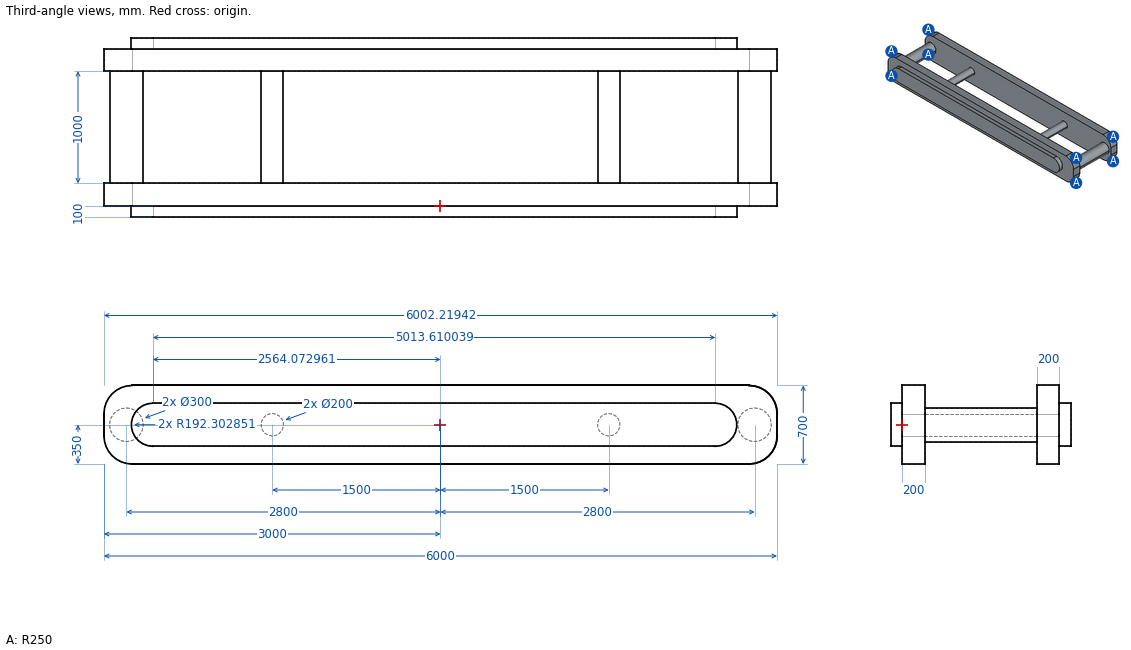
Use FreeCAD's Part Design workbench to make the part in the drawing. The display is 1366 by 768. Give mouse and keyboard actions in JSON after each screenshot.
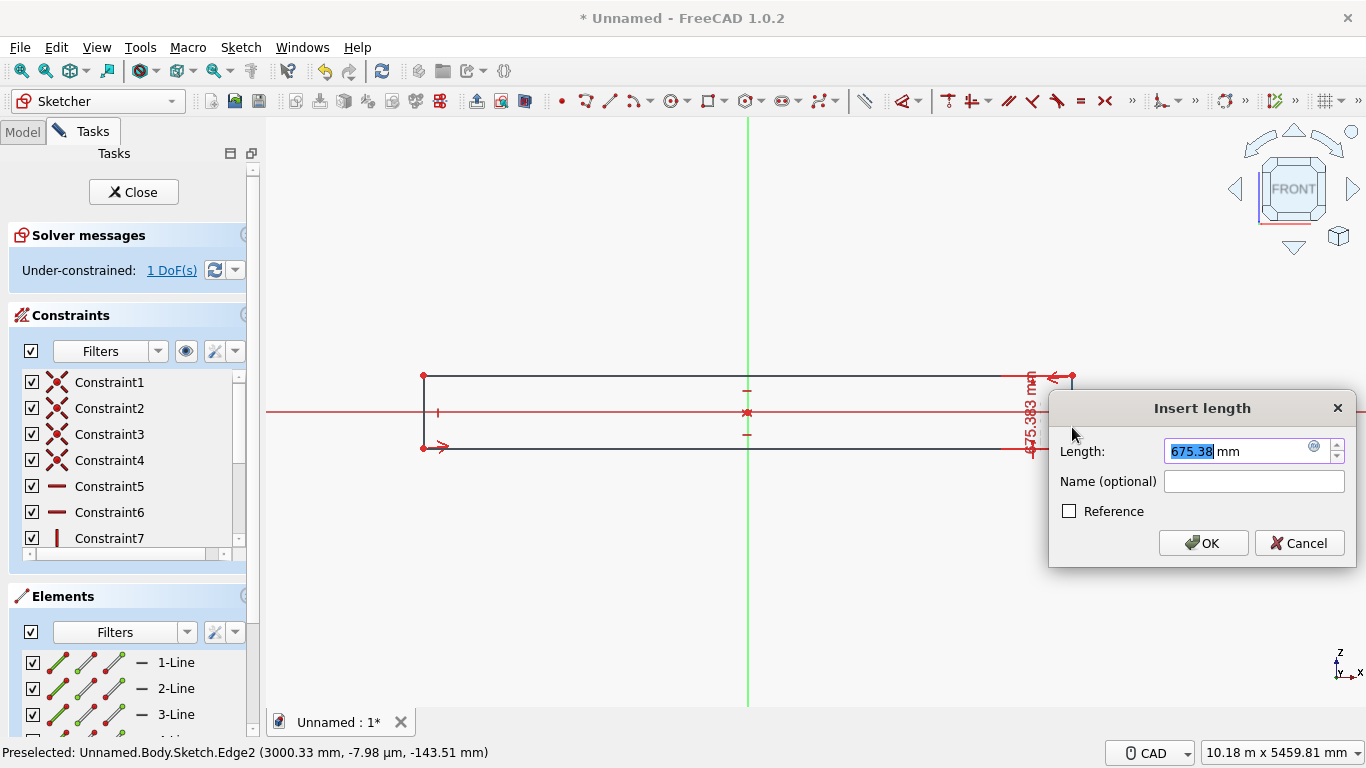
{"action": "type", "text": "700"}
{"action": "key", "text": "Return"}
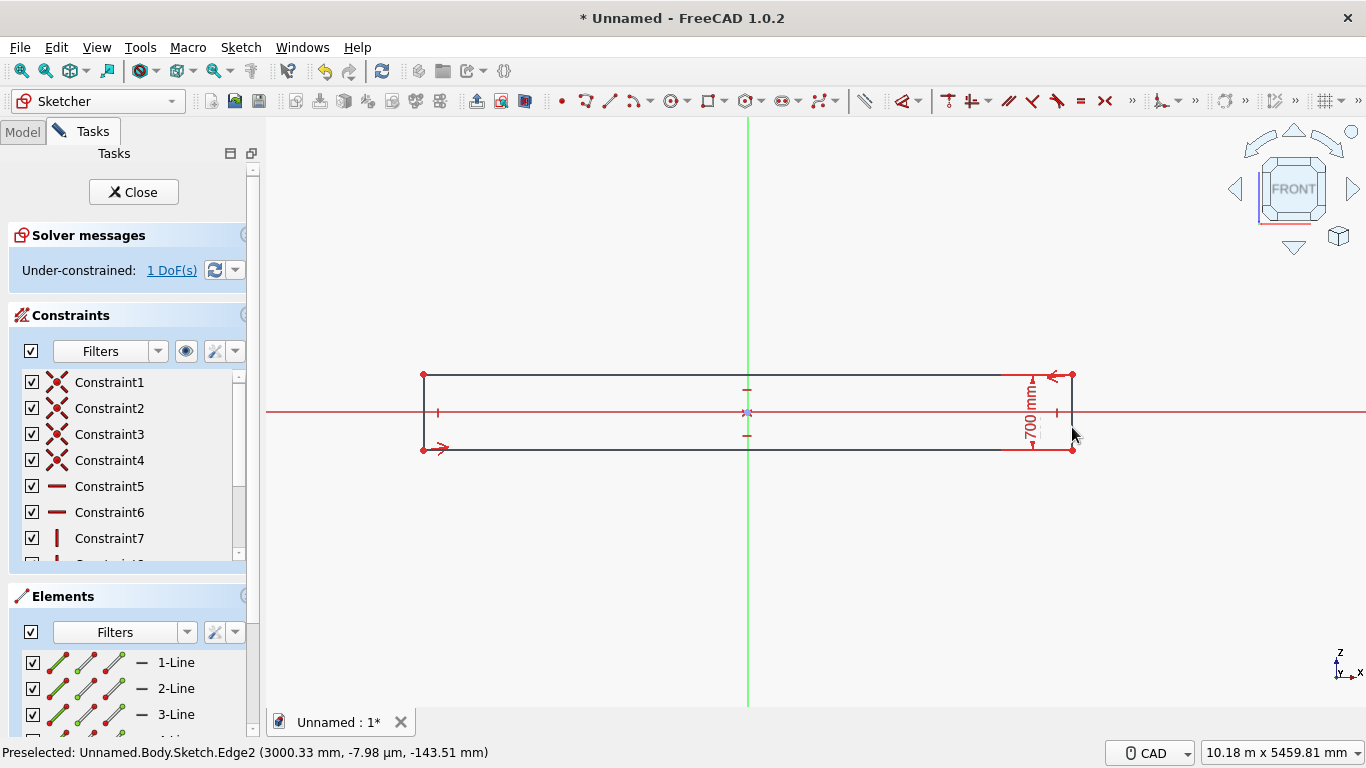
{"action": "left_click", "coordinate": [618, 450]}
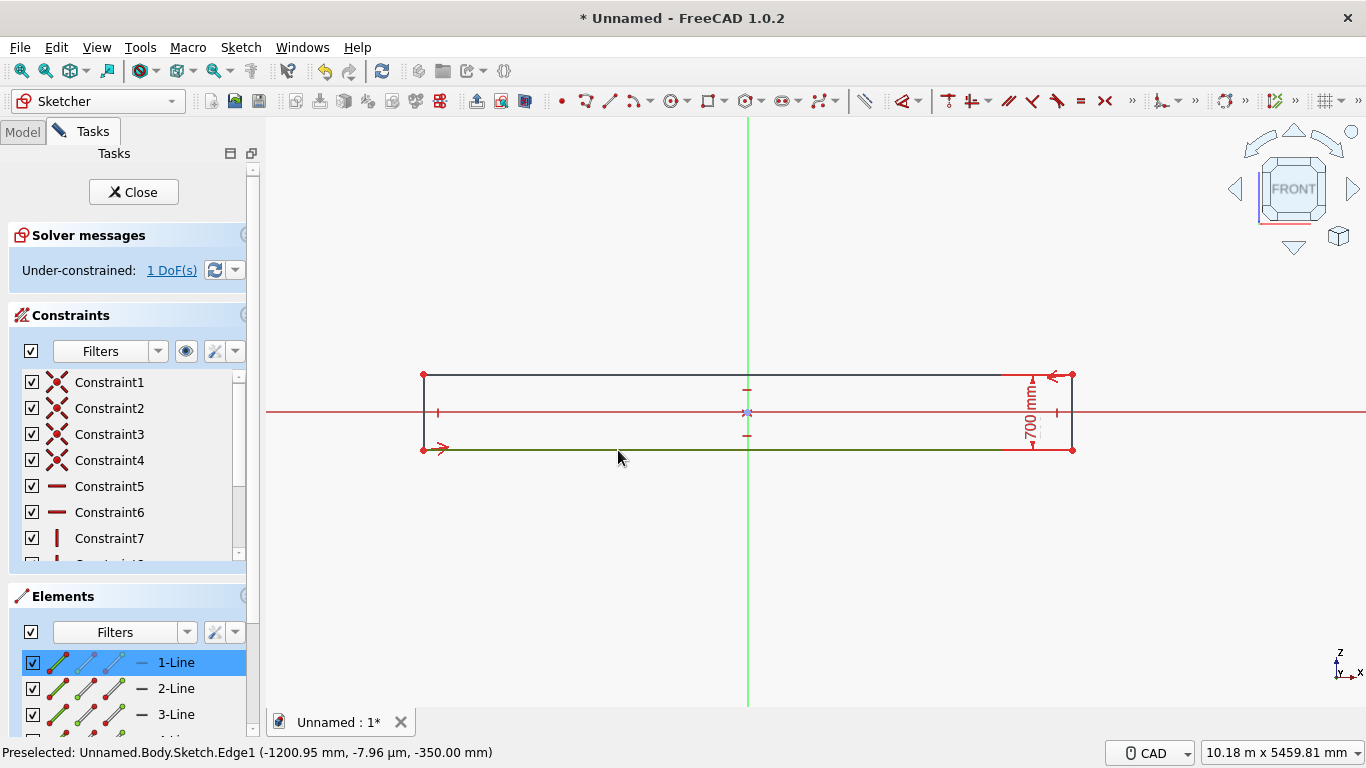
{"action": "key", "text": "l"}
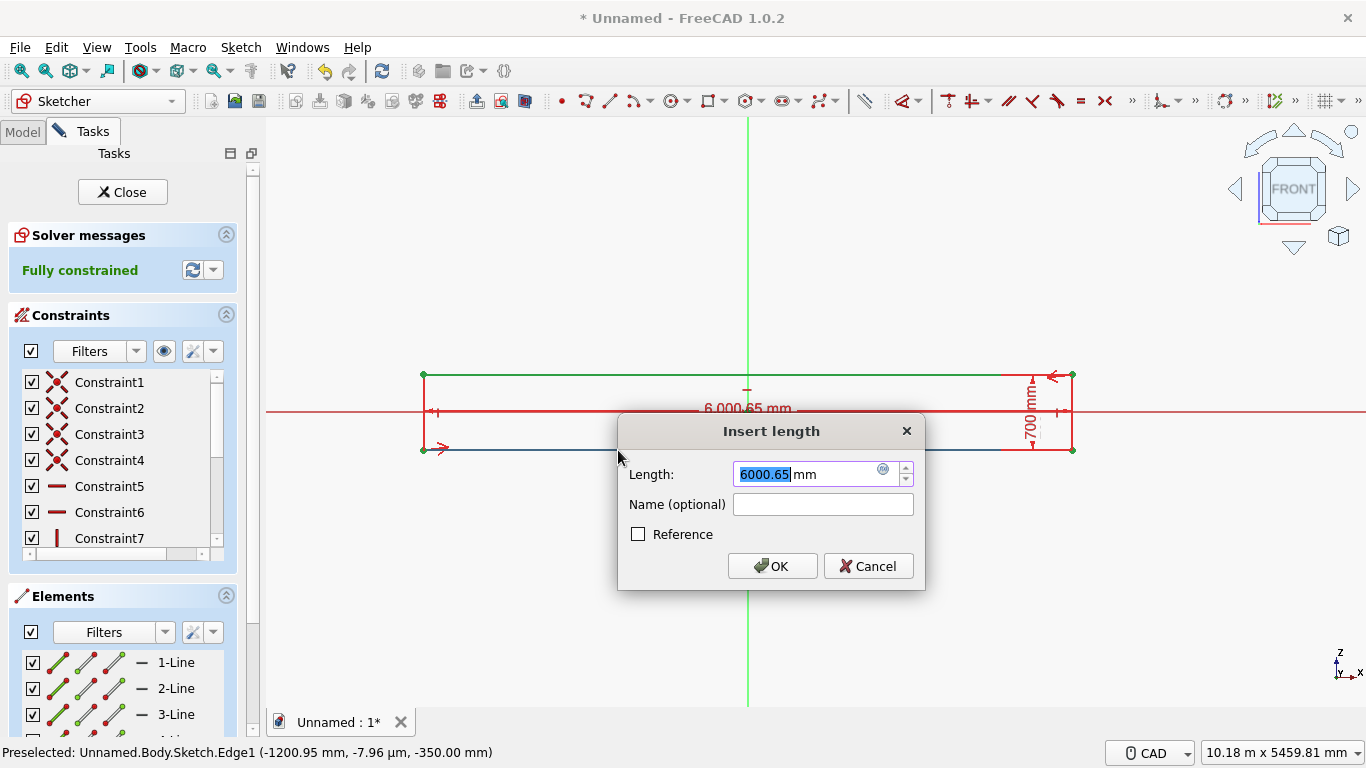
{"action": "type", "text": "6000"}
{"action": "key", "text": "Return"}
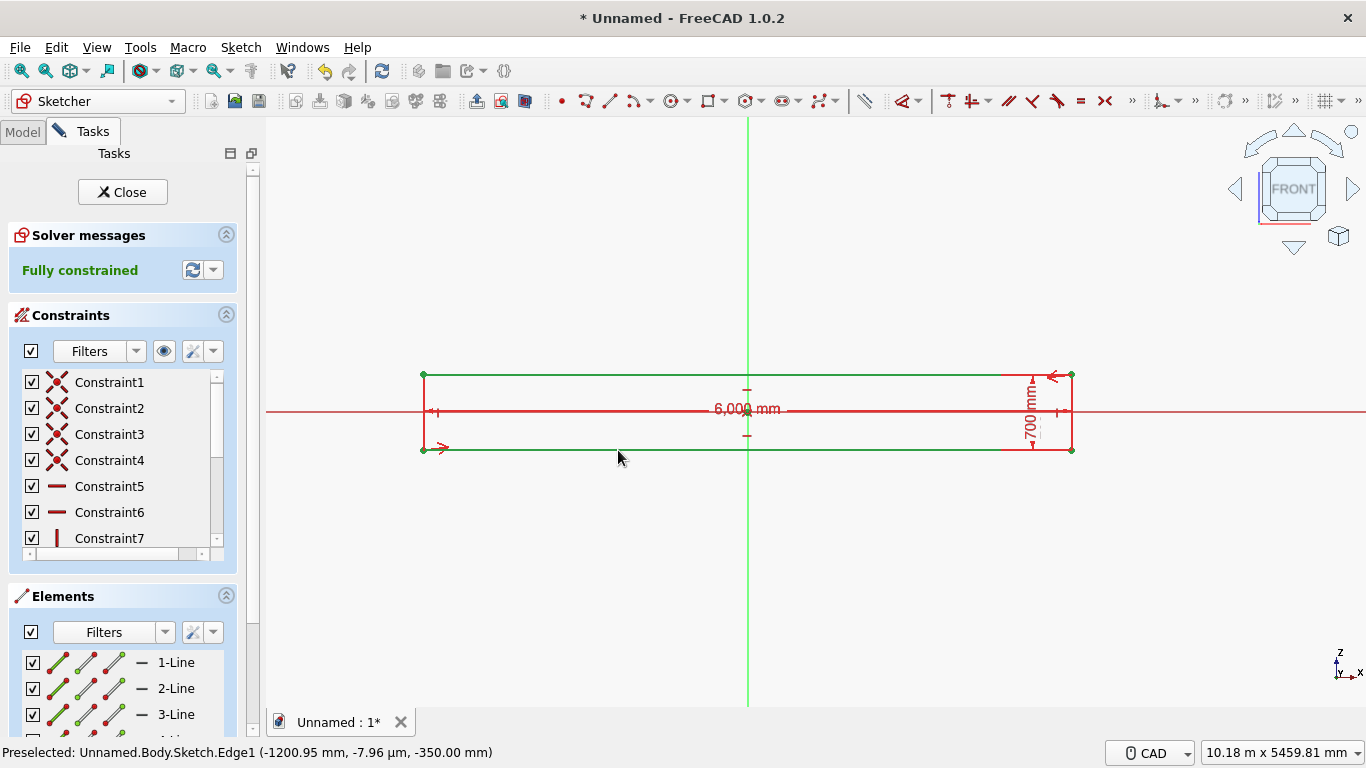
{"action": "left_click", "coordinate": [123, 192]}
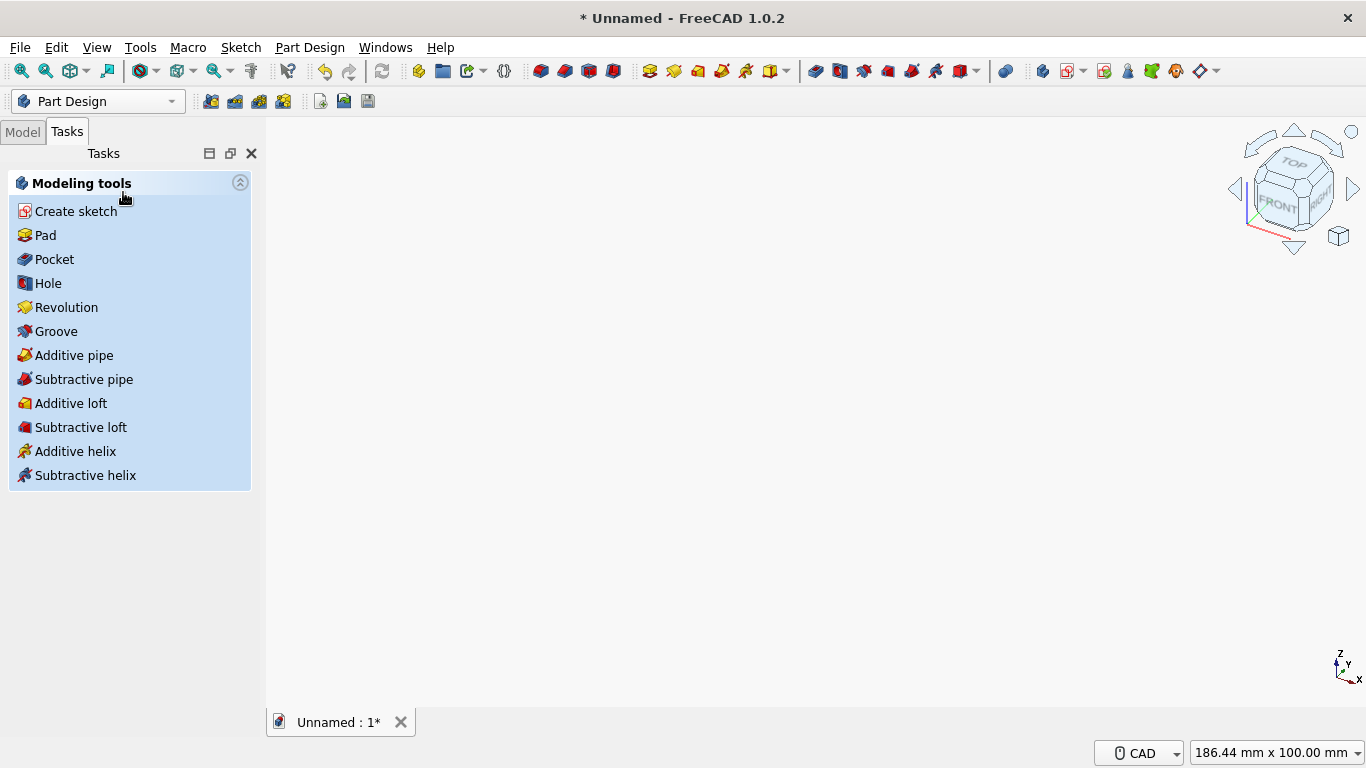
{"action": "left_click", "coordinate": [650, 72]}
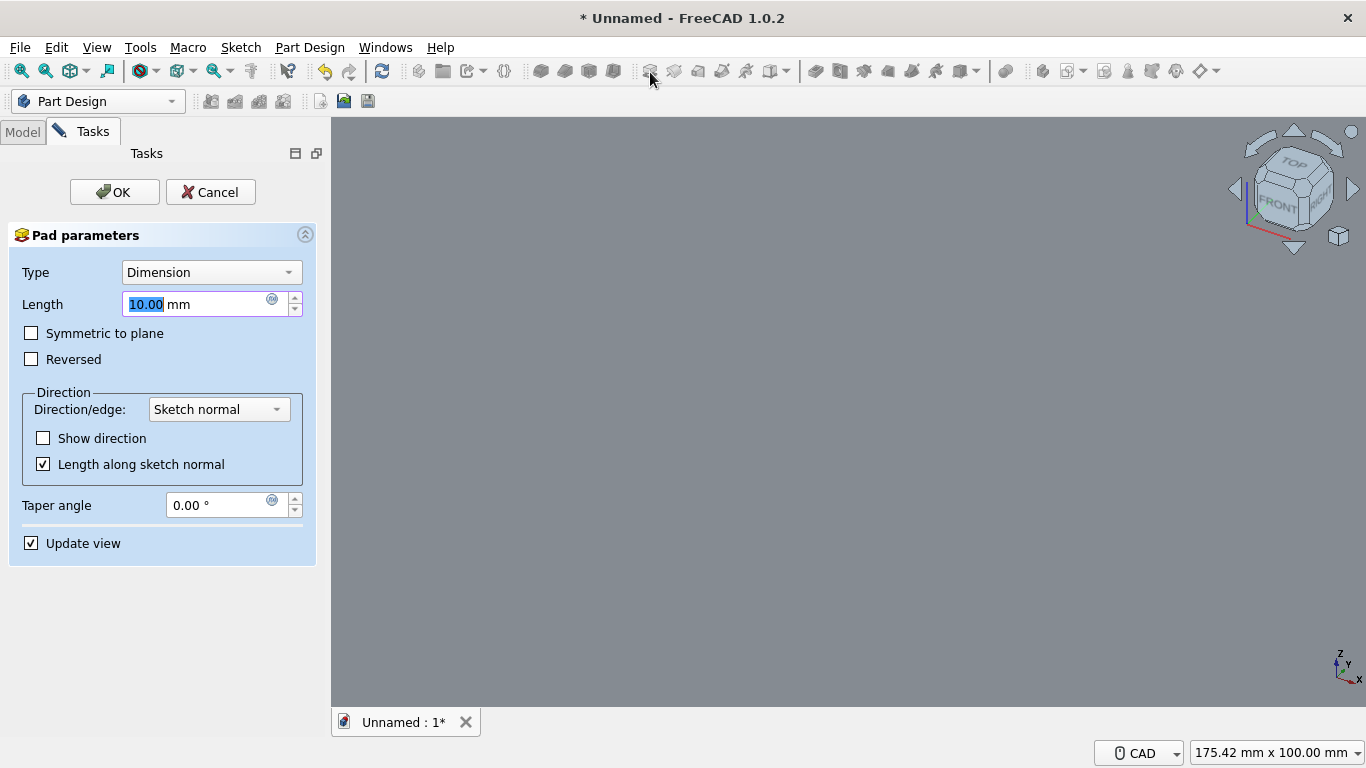
{"action": "type", "text": "200"}
{"action": "key", "text": "Tab"}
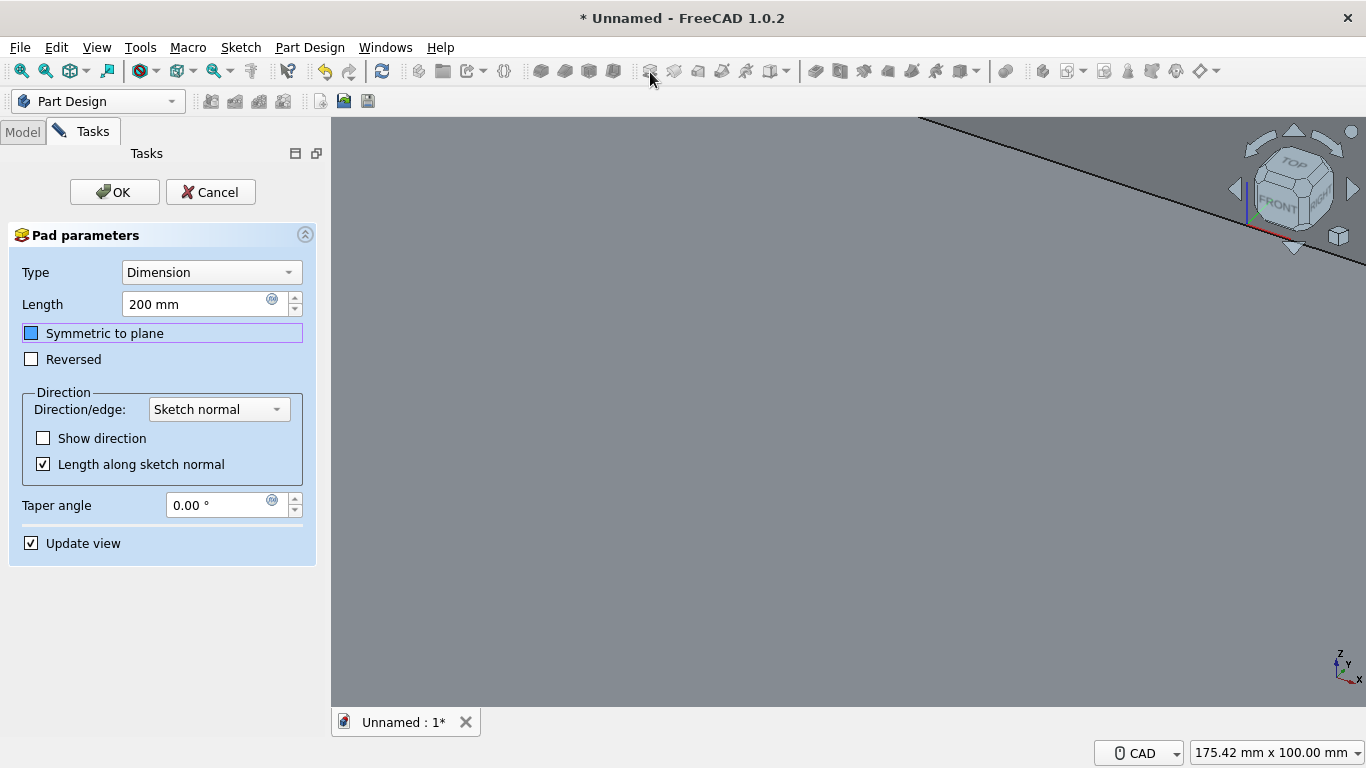
{"action": "left_click", "coordinate": [30, 359]}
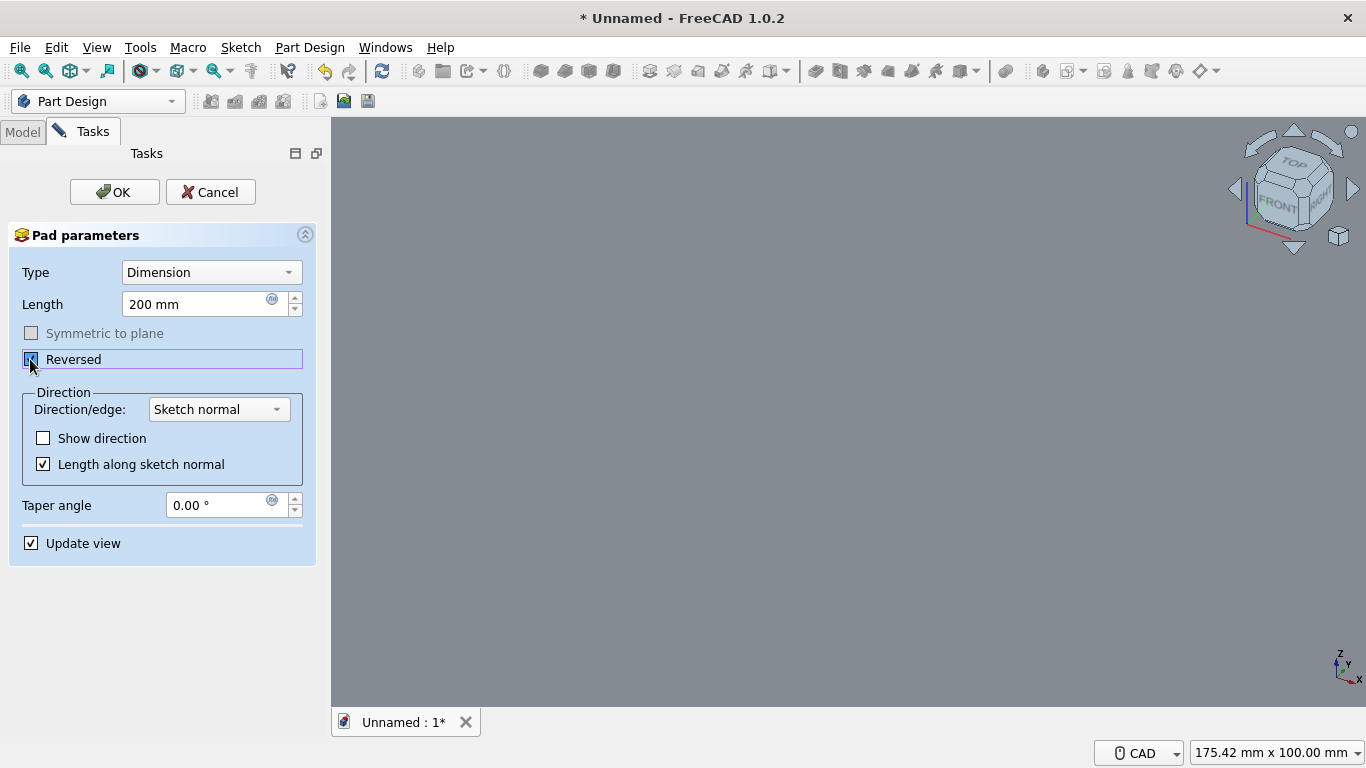
{"action": "left_click", "coordinate": [115, 192]}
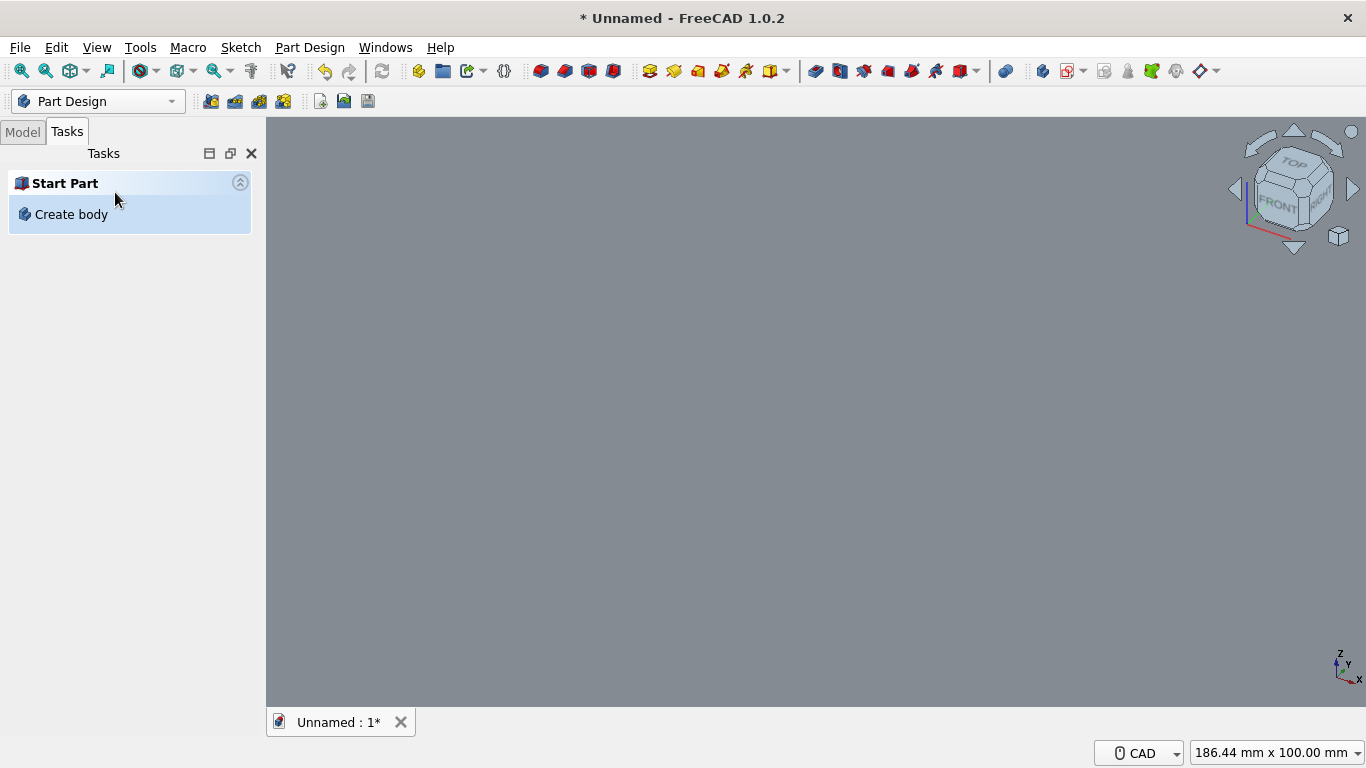
{"action": "left_click", "coordinate": [22, 72]}